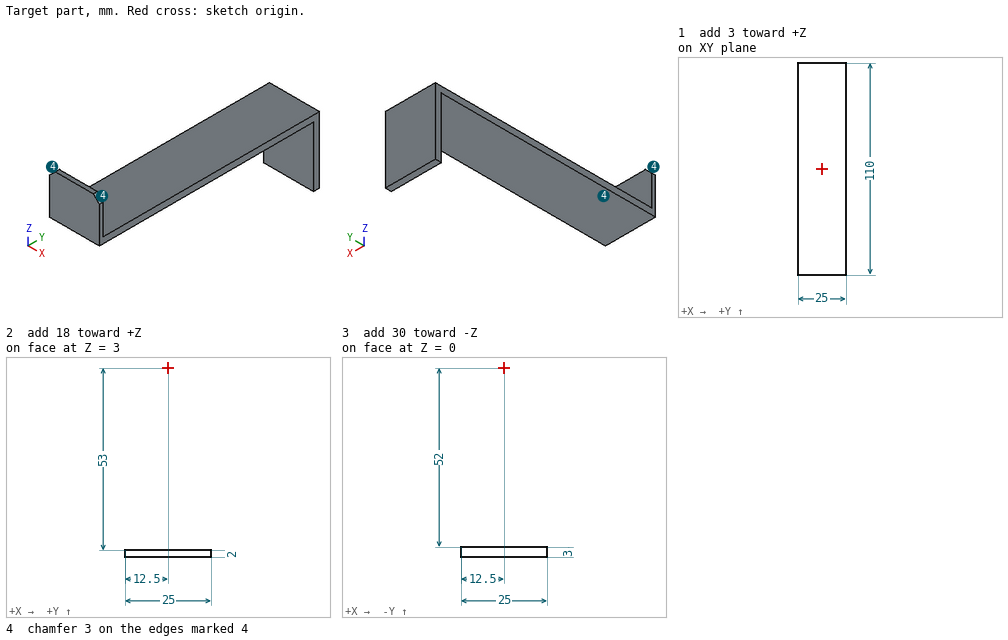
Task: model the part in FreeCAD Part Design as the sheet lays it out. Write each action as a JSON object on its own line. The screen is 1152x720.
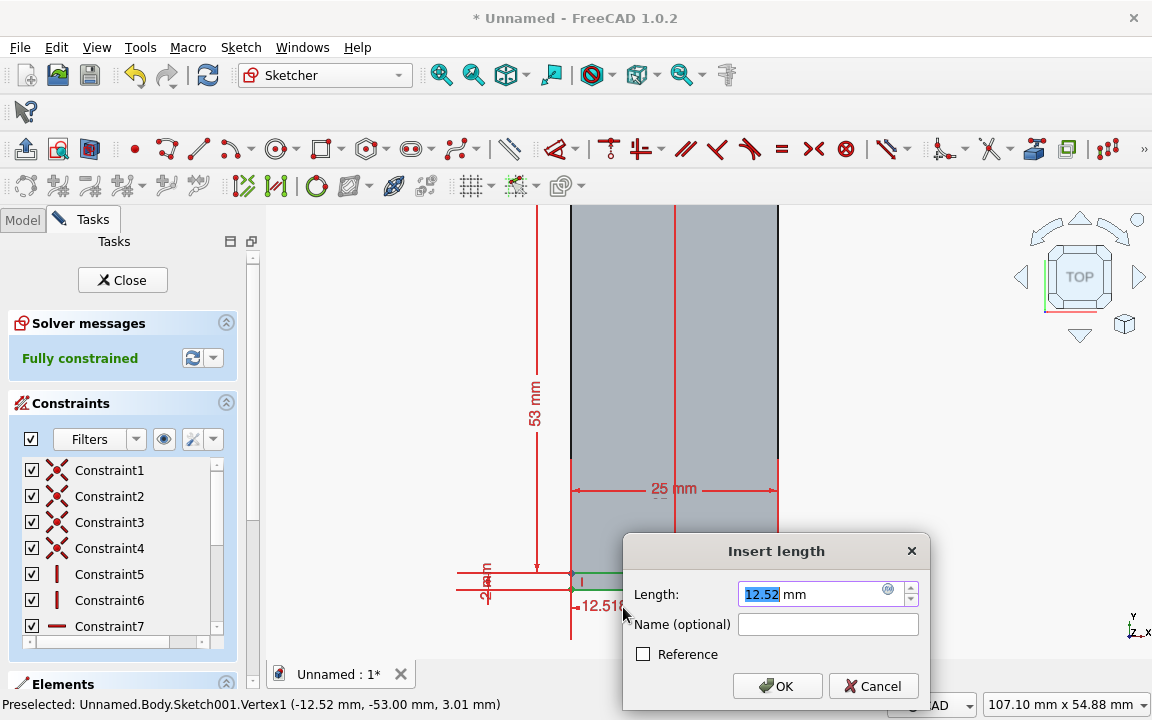
{"action": "type", "text": "12.5"}
{"action": "key", "text": "Return"}
{"action": "key", "text": "Escape"}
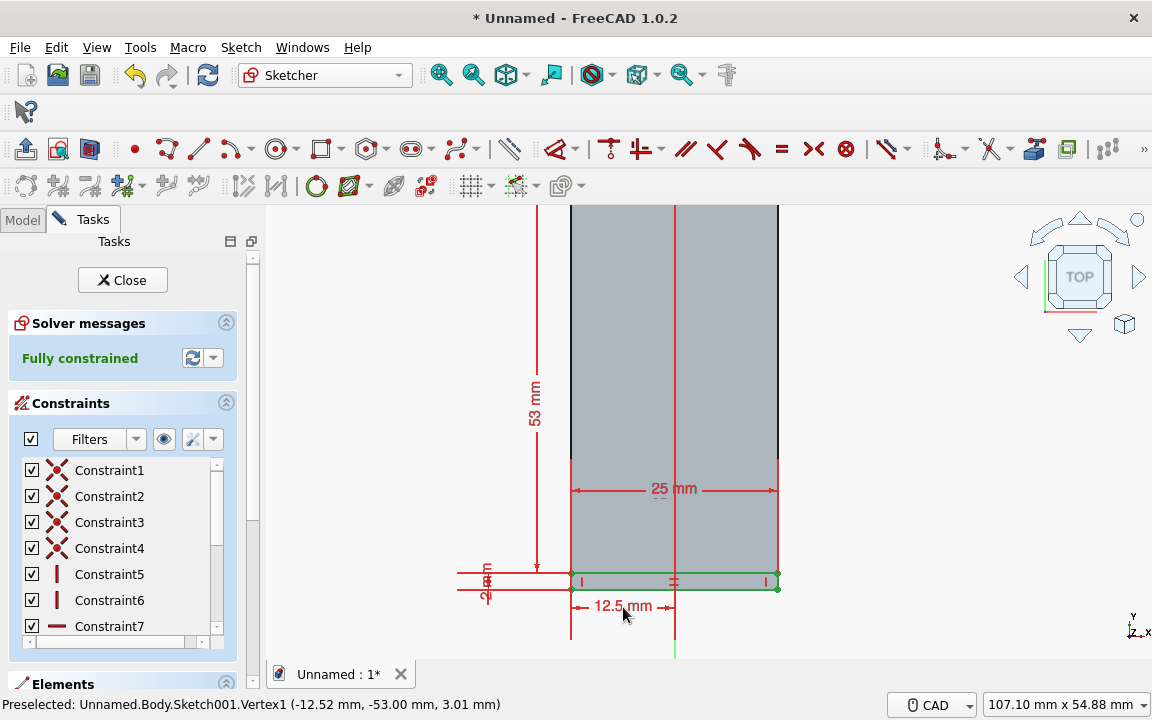
{"action": "left_click", "coordinate": [123, 280]}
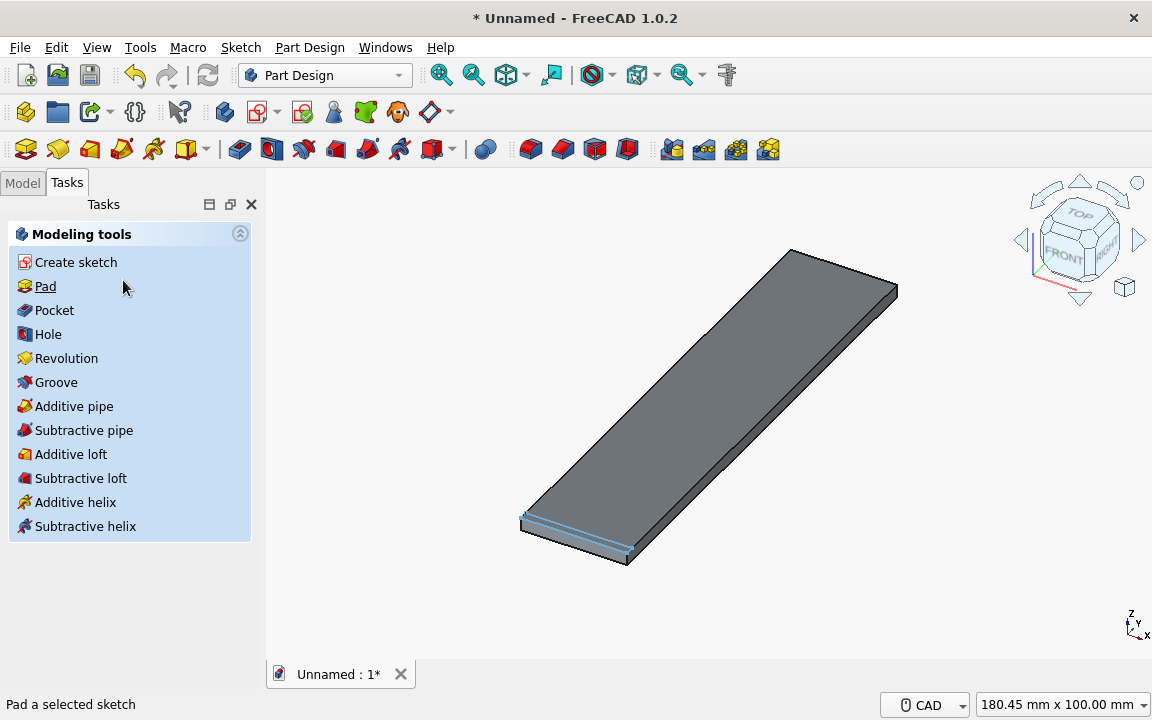
{"action": "left_click", "coordinate": [26, 150]}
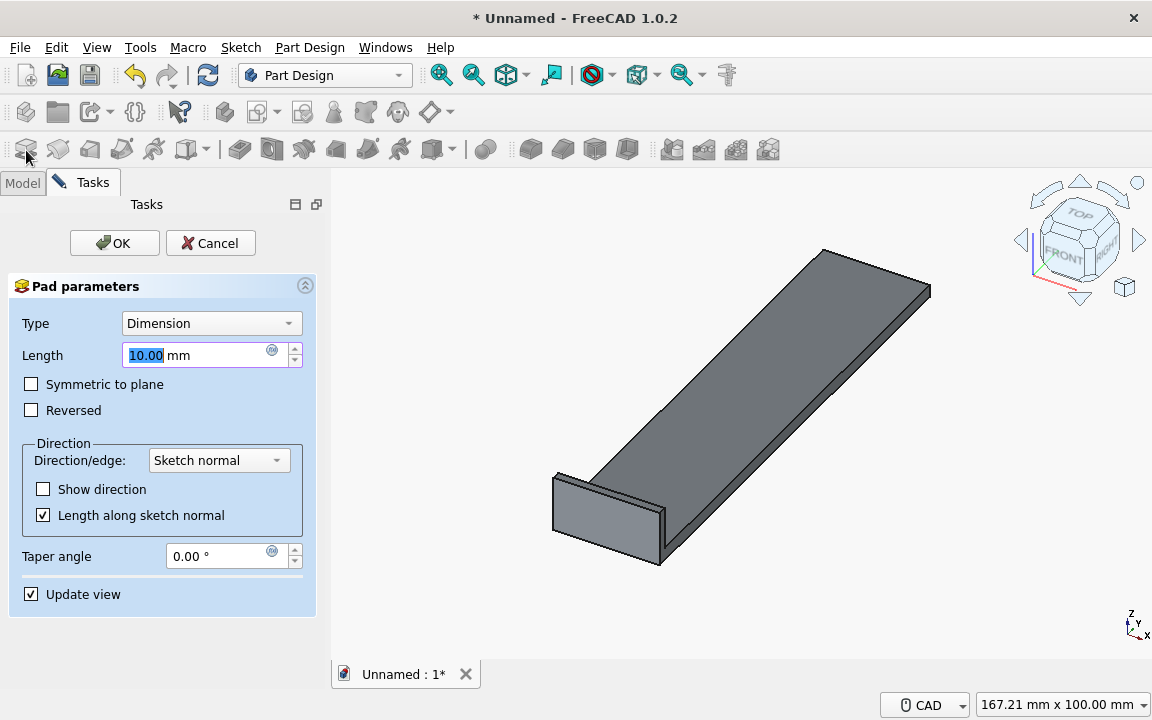
{"action": "type", "text": "18"}
{"action": "key", "text": "Tab"}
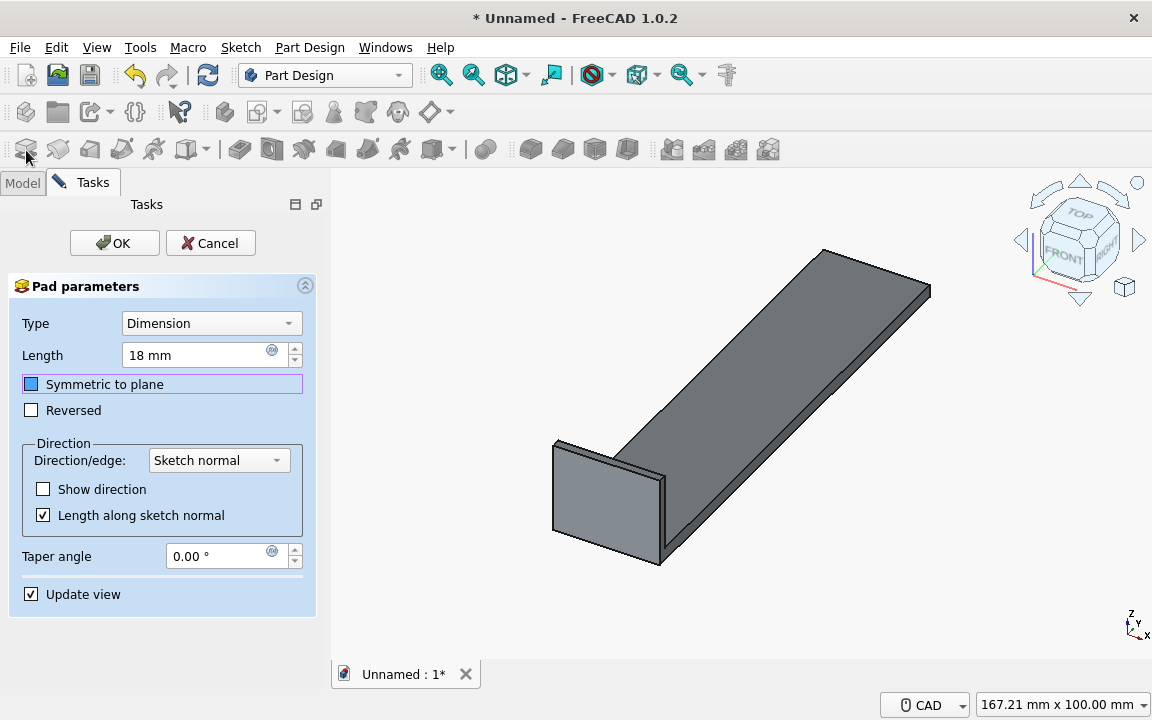
{"action": "left_click", "coordinate": [115, 243]}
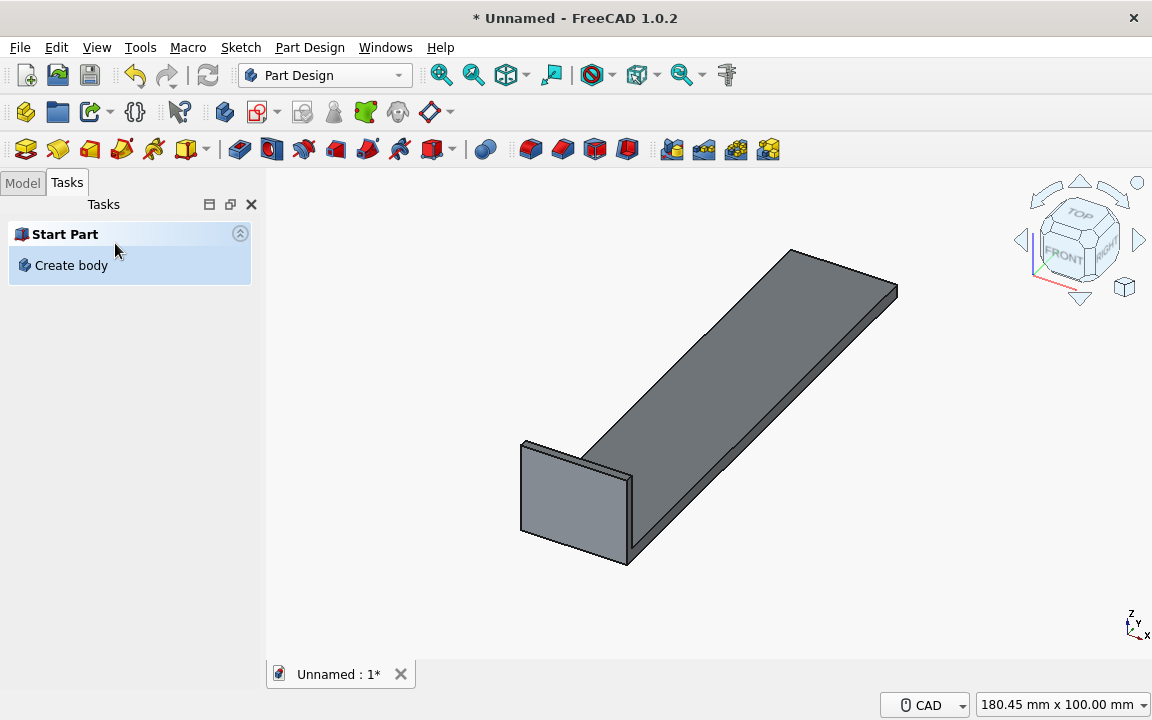
{"action": "key", "text": "5"}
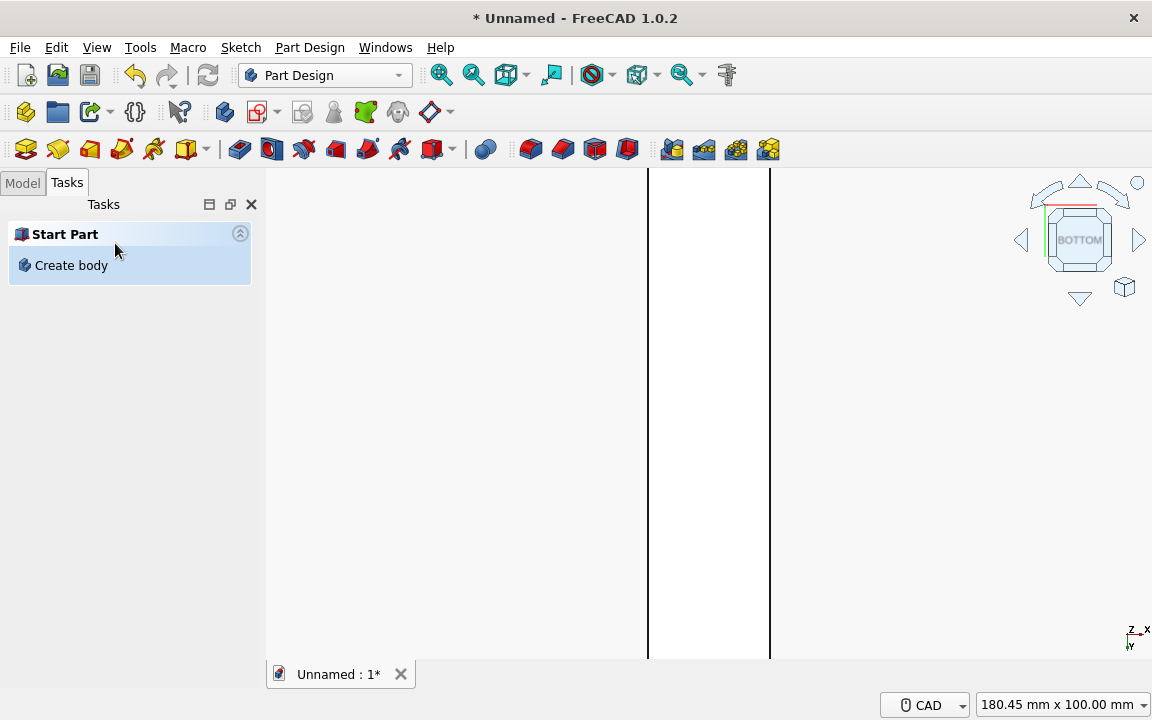
{"action": "key", "text": "v f"}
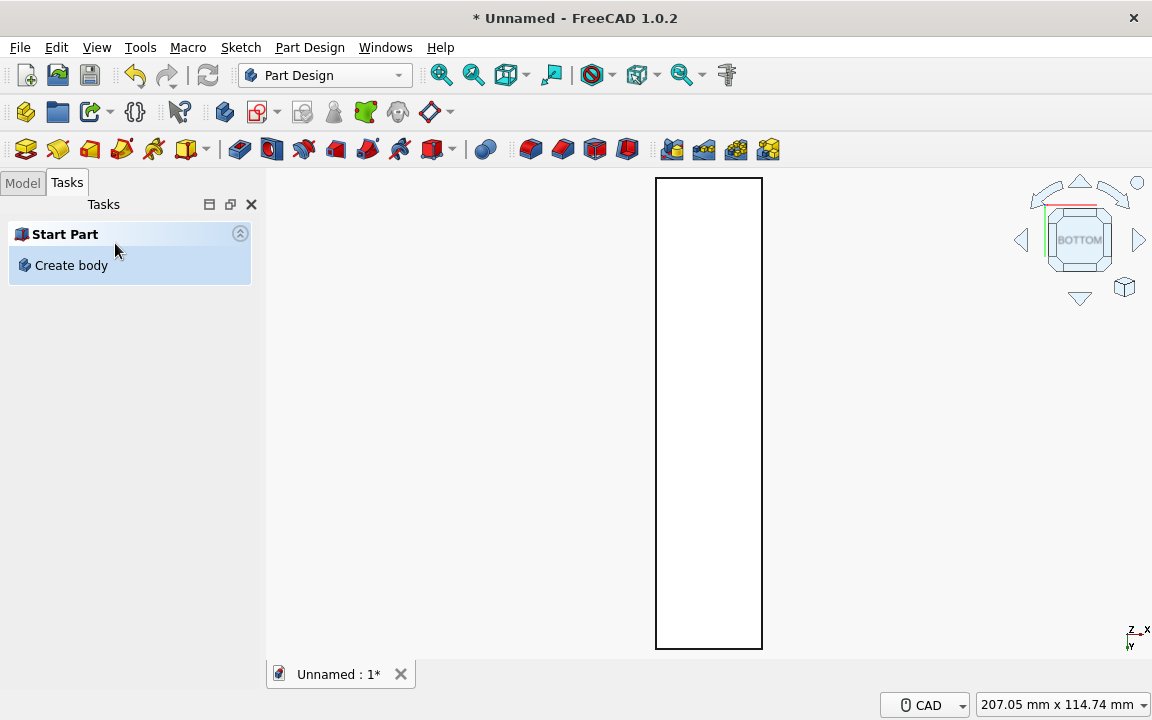
{"action": "left_click", "coordinate": [709, 547]}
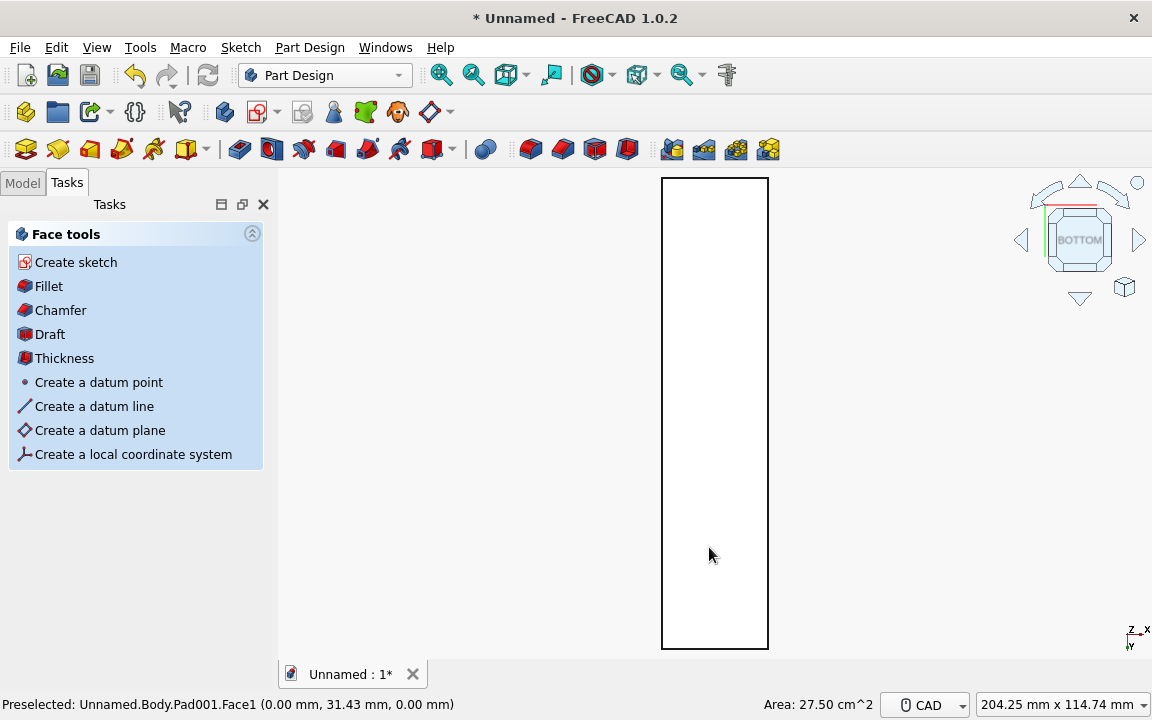
{"action": "left_click", "coordinate": [258, 112]}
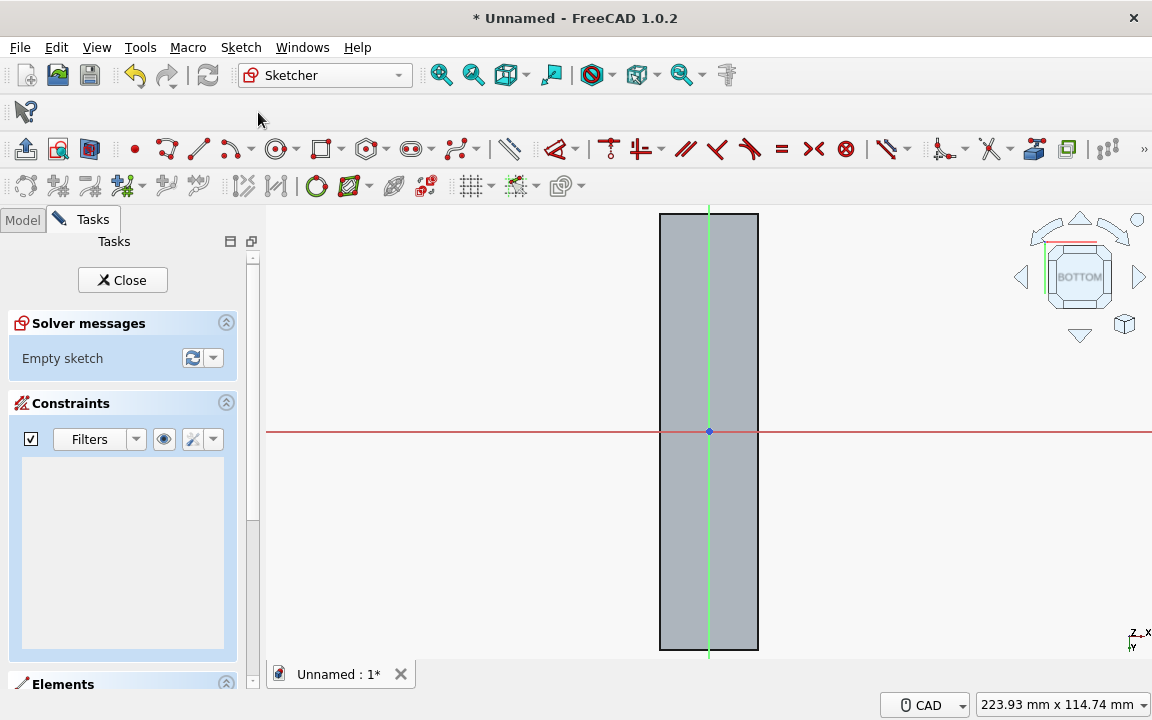
{"action": "scroll", "coordinate": [331, 233], "scroll_direction": "down", "scroll_amount": 1}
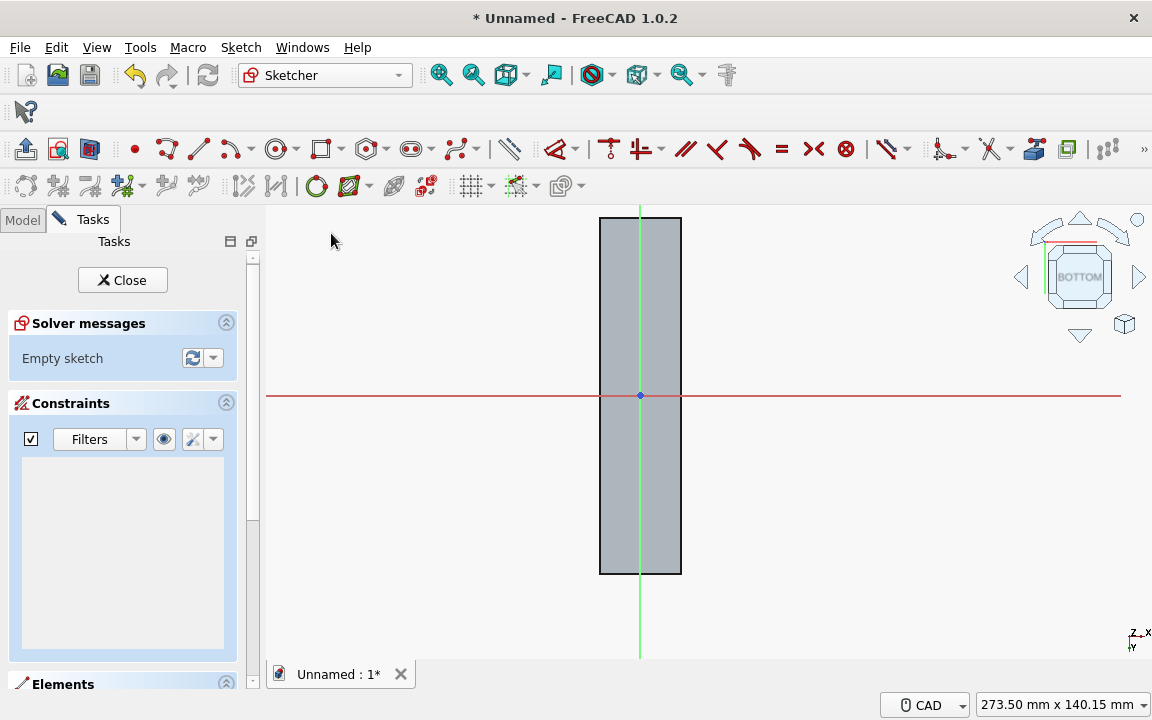
{"action": "scroll", "coordinate": [640, 593], "scroll_direction": "up", "scroll_amount": 2}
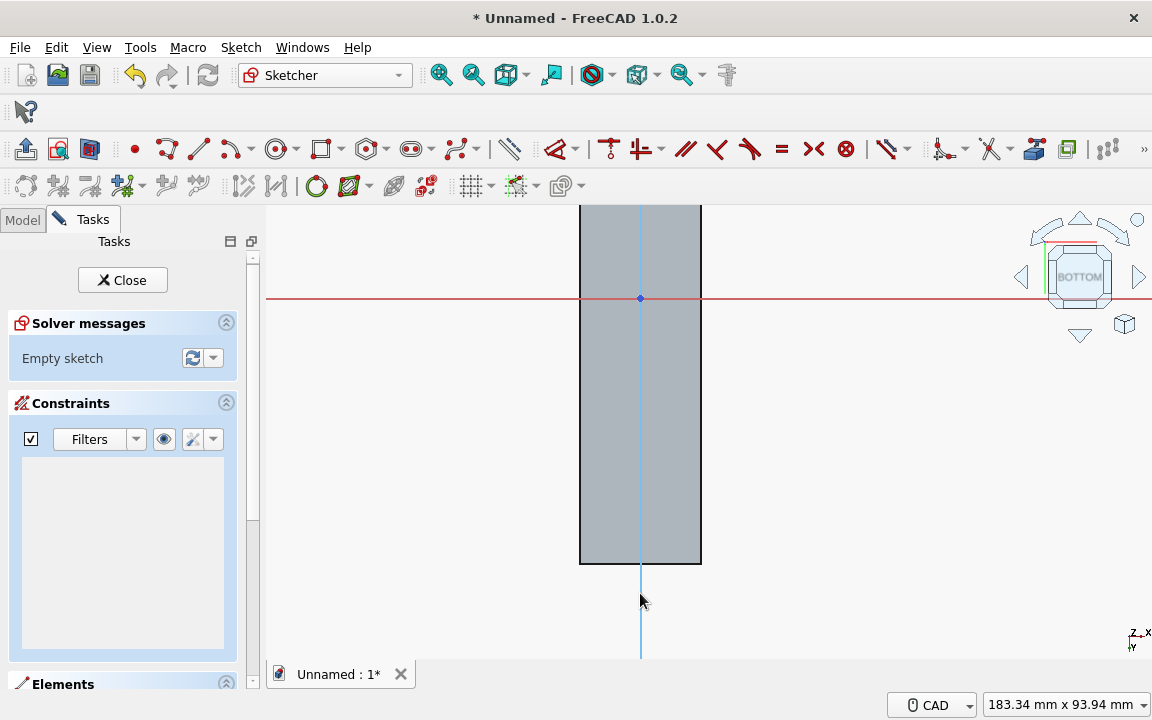
{"action": "key", "text": "g r"}